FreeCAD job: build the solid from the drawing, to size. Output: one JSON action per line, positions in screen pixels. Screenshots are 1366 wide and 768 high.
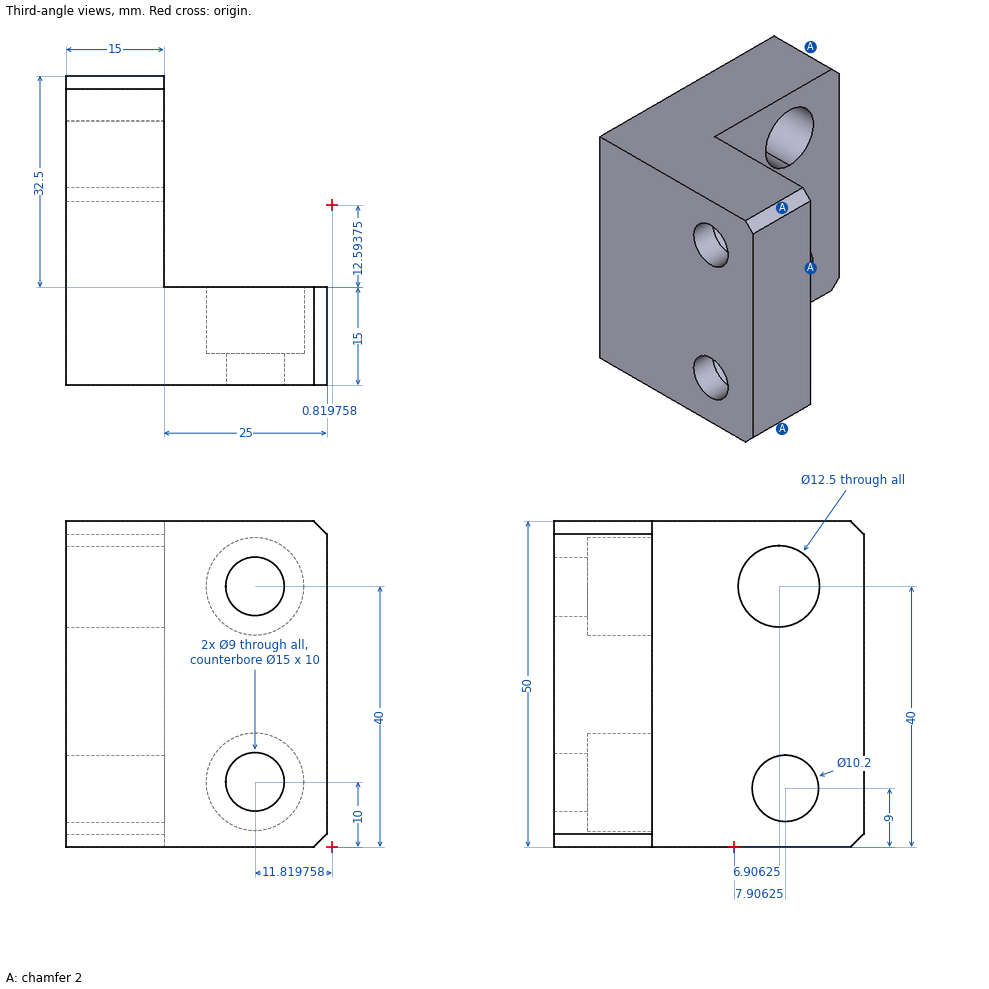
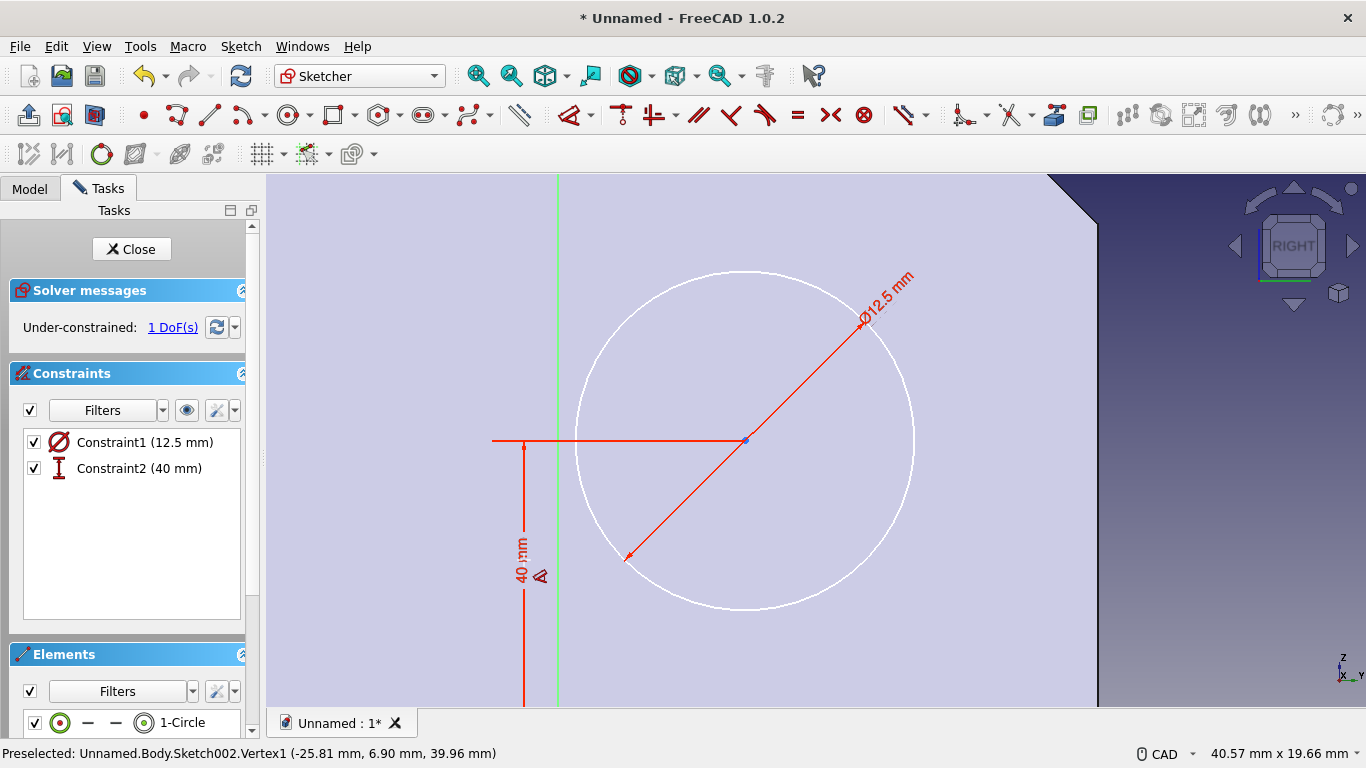
{"action": "left_click", "coordinate": [745, 441]}
{"action": "left_click", "coordinate": [651, 407]}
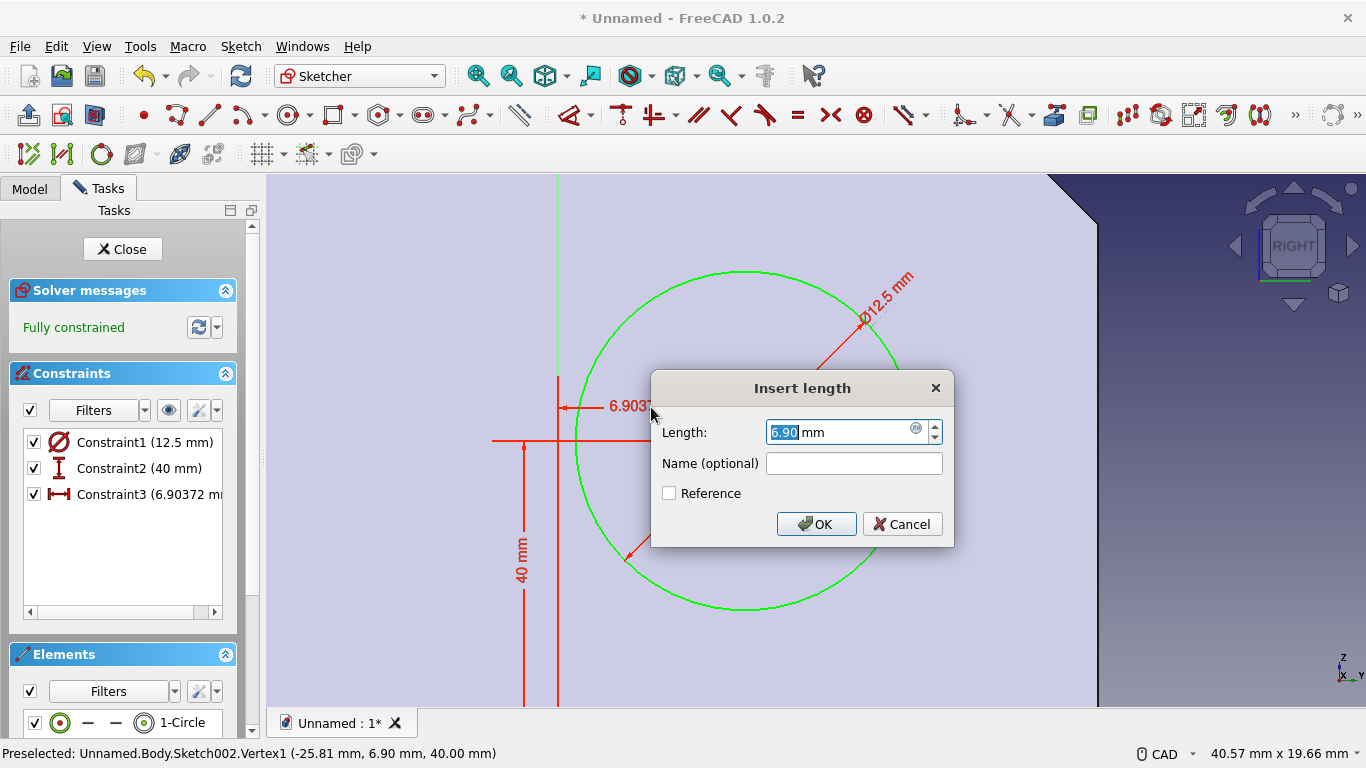
{"action": "type", "text": "6.90625"}
{"action": "key", "text": "Return"}
{"action": "key", "text": "Escape"}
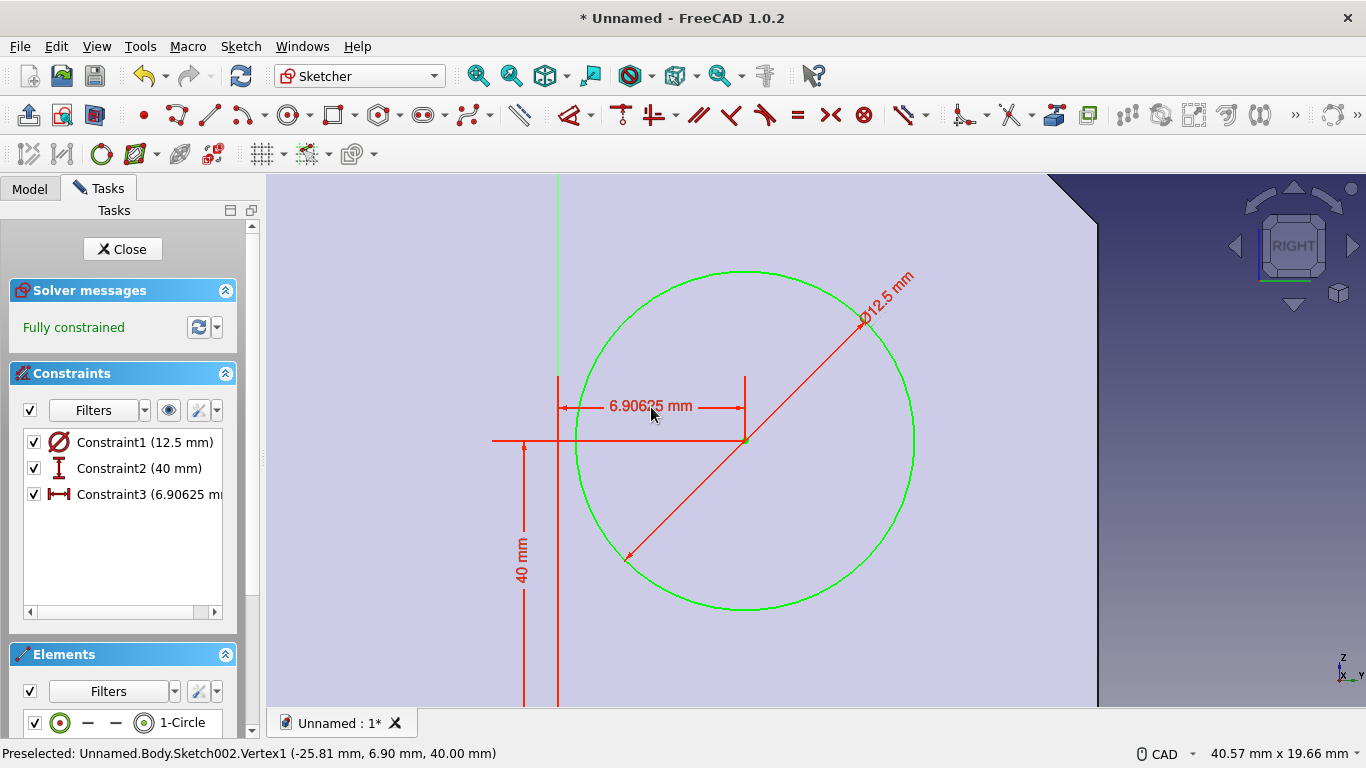
{"action": "left_click", "coordinate": [123, 249]}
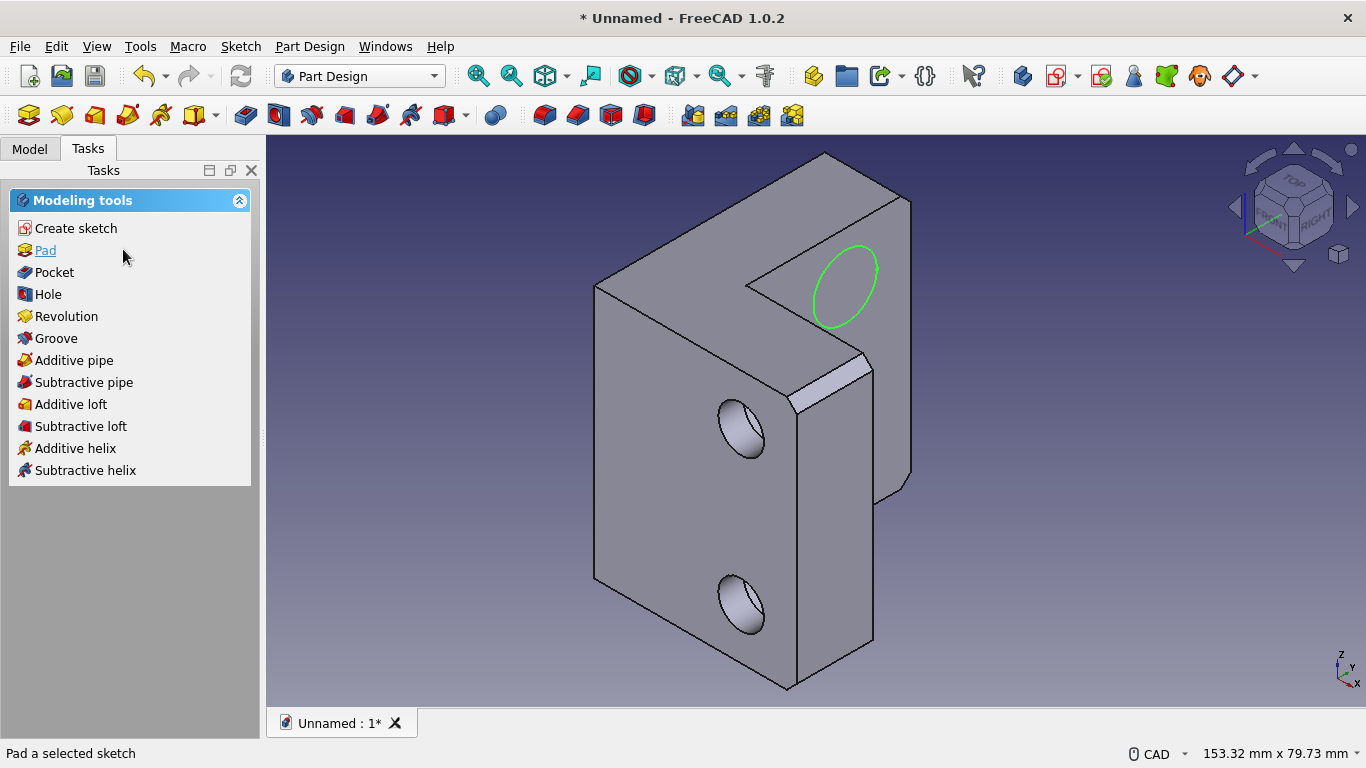
{"action": "left_click", "coordinate": [279, 116]}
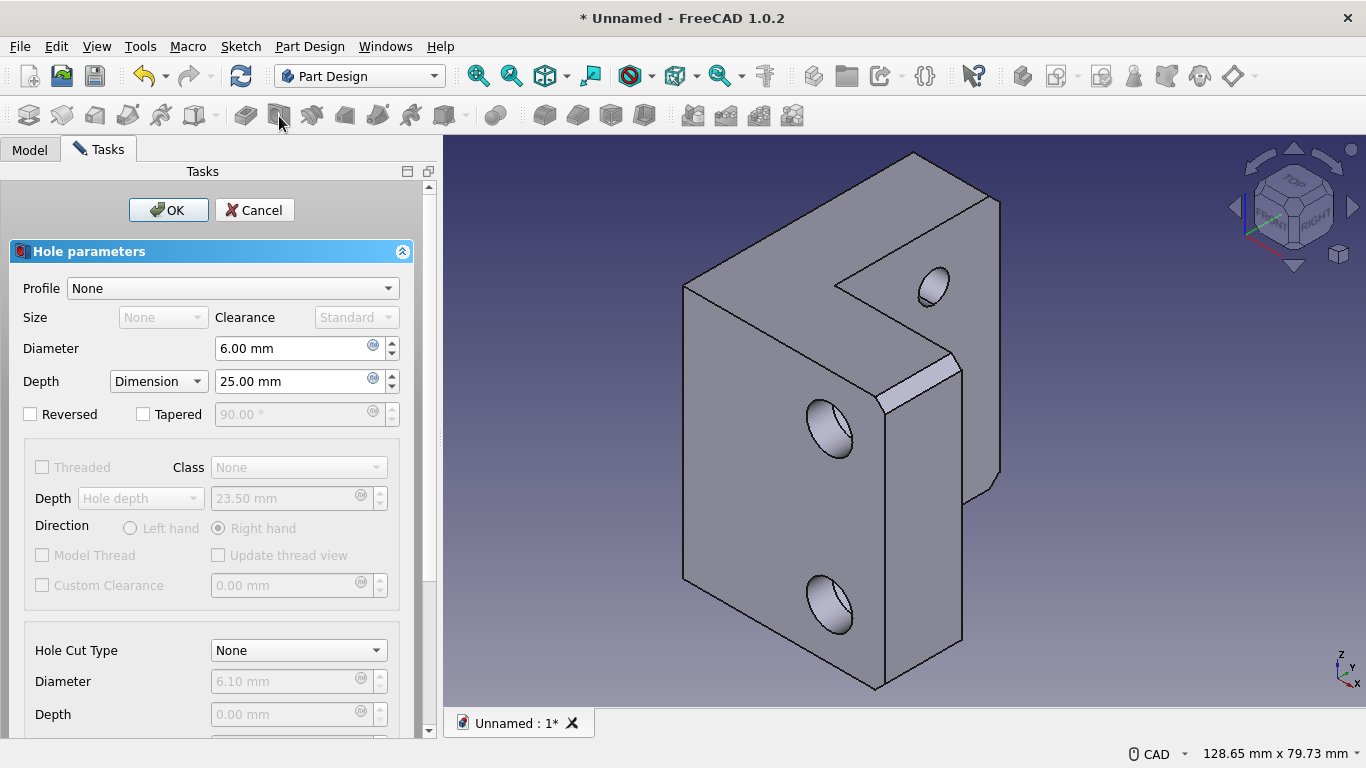
{"action": "triple_click", "coordinate": [300, 348]}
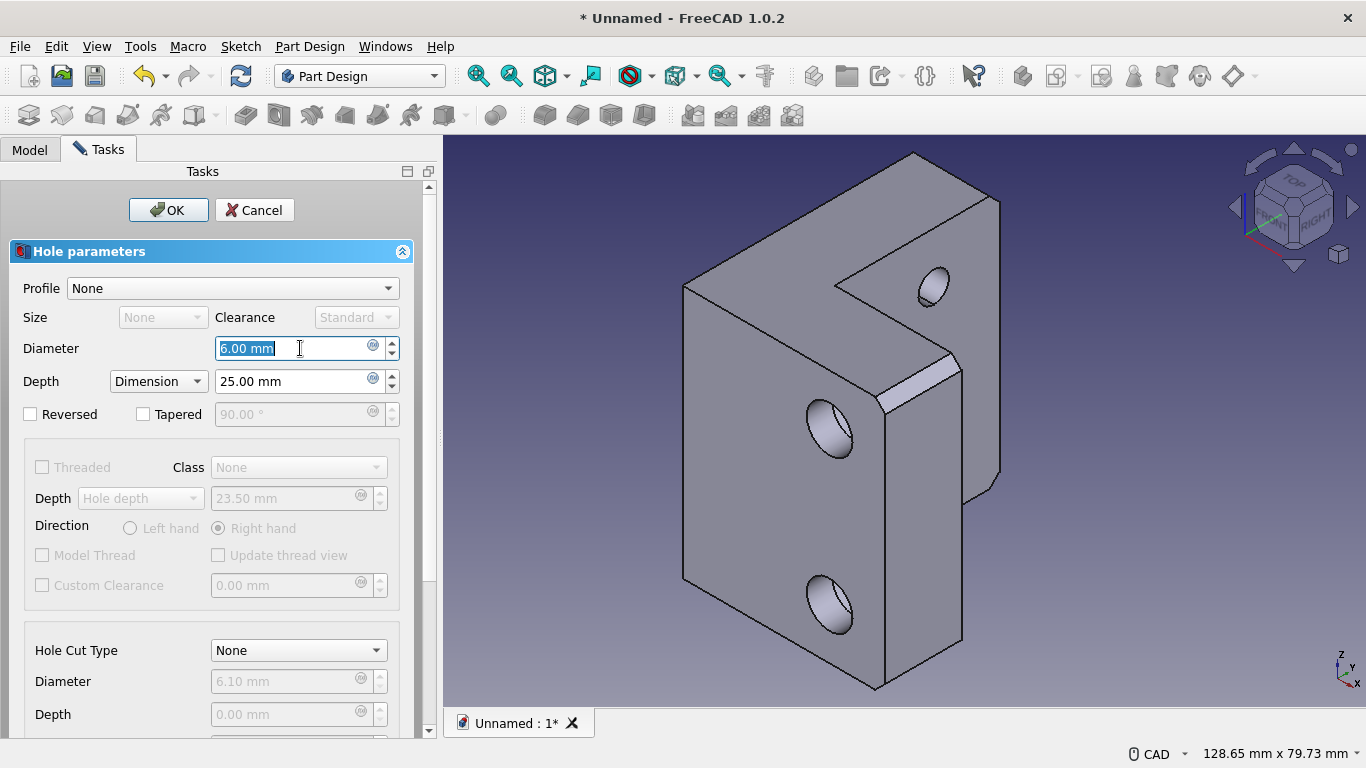
{"action": "type", "text": "12.5"}
{"action": "key", "text": "Tab"}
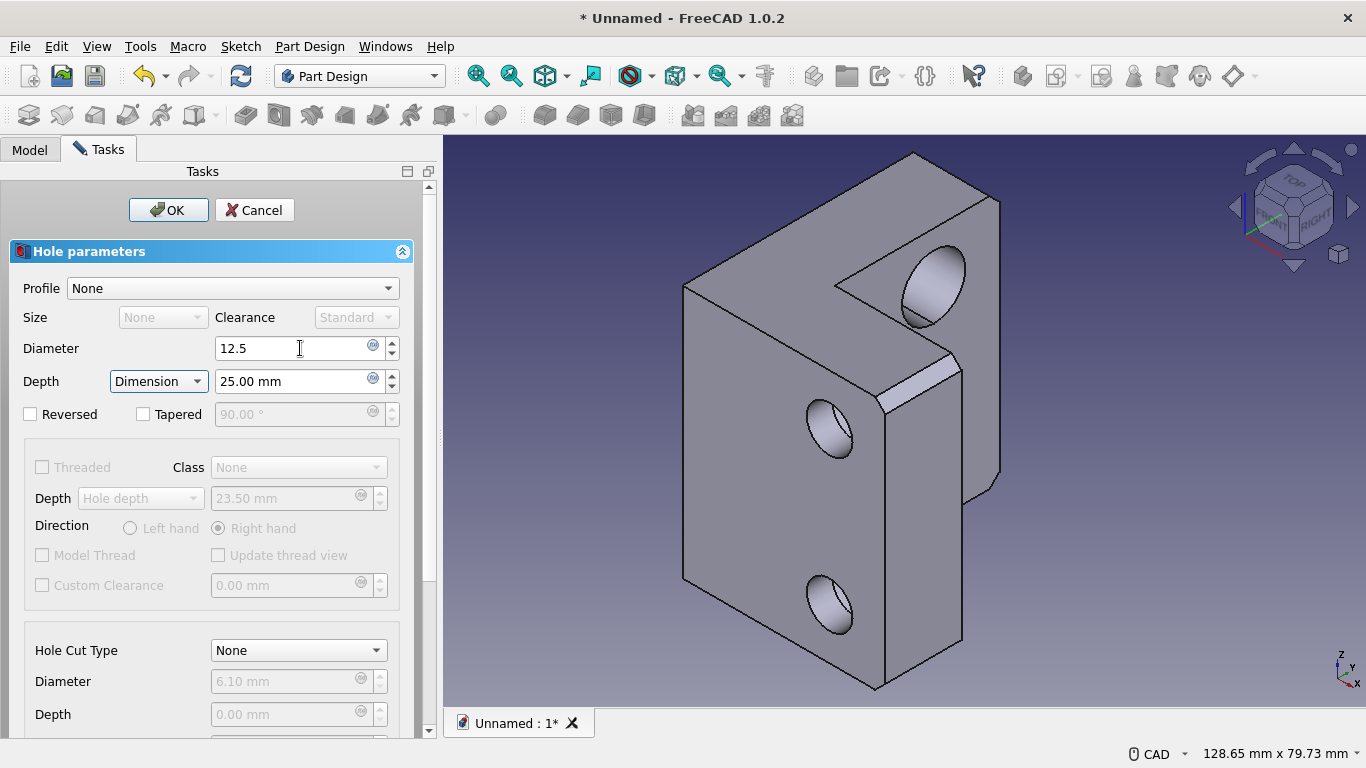
{"action": "left_click", "coordinate": [160, 382]}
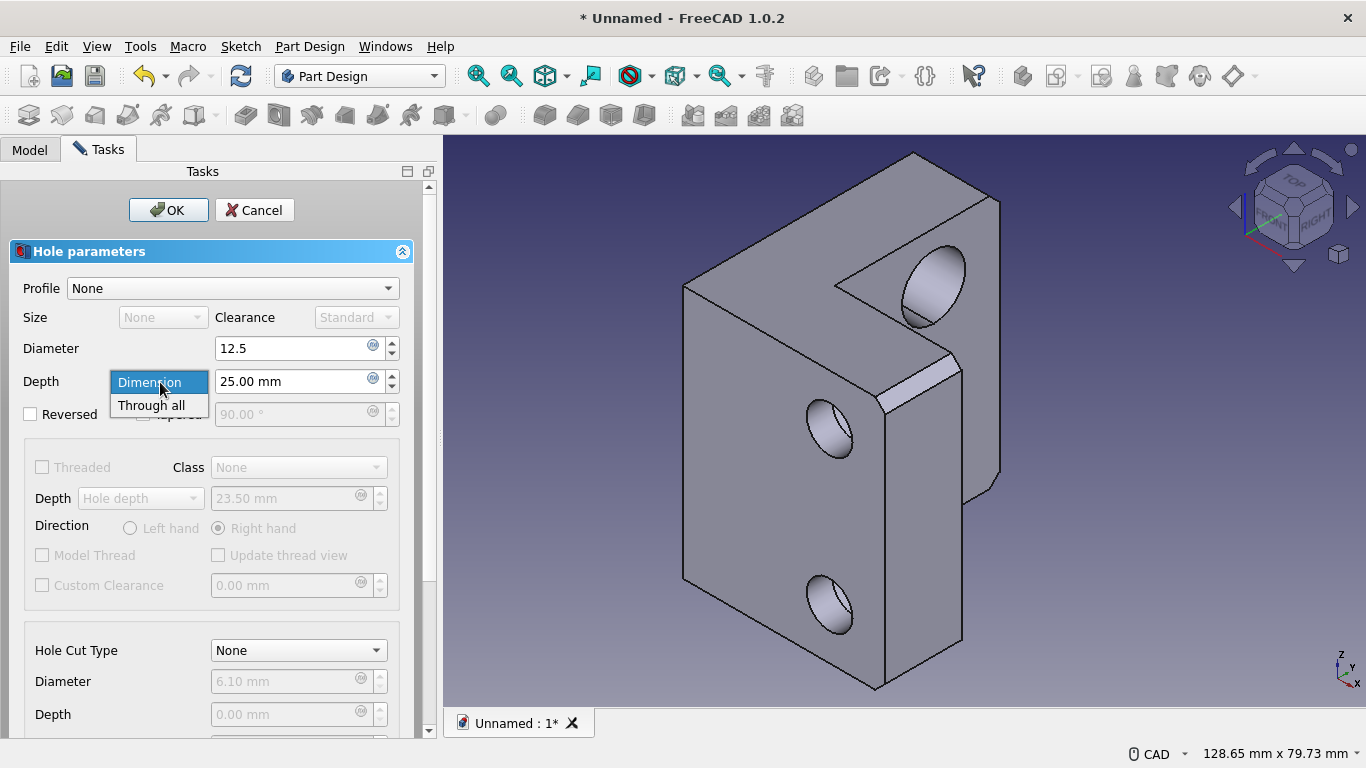
{"action": "left_click", "coordinate": [158, 406]}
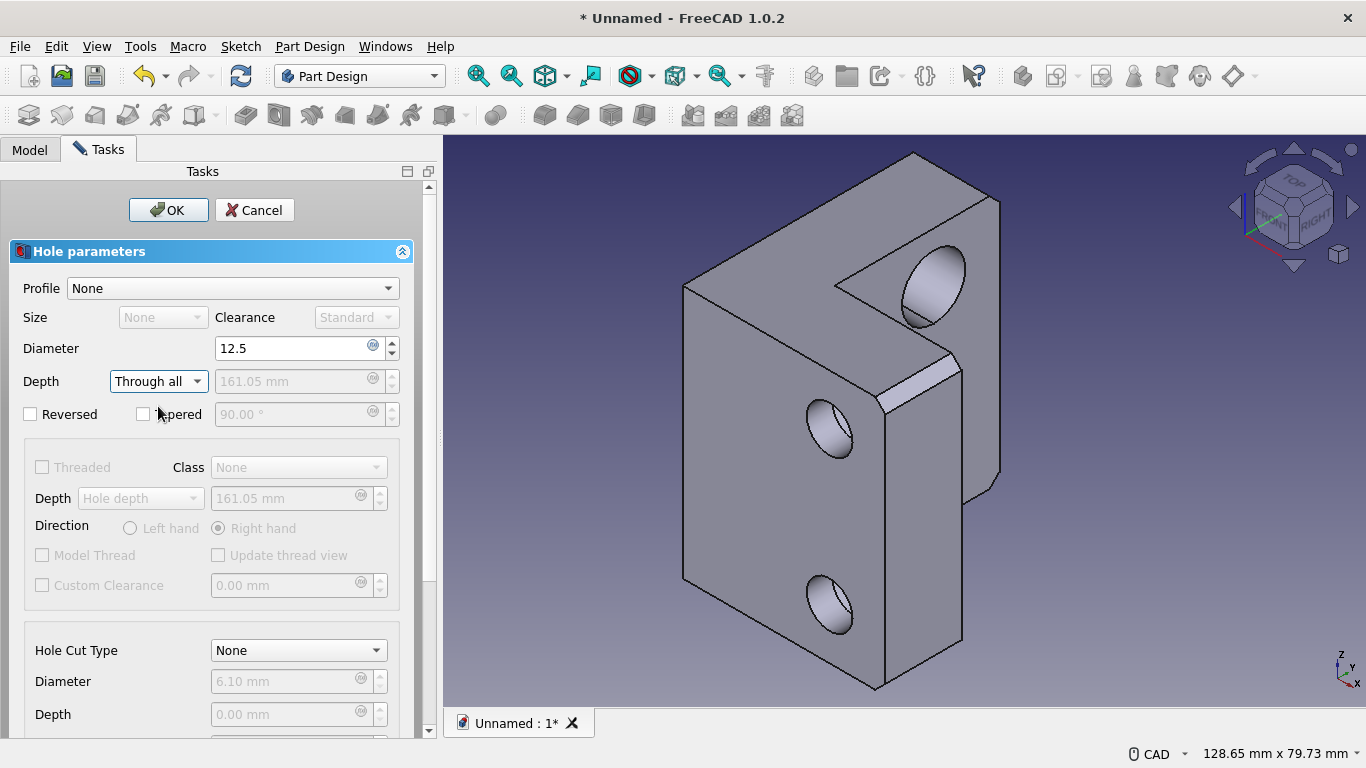
{"action": "left_click", "coordinate": [169, 210]}